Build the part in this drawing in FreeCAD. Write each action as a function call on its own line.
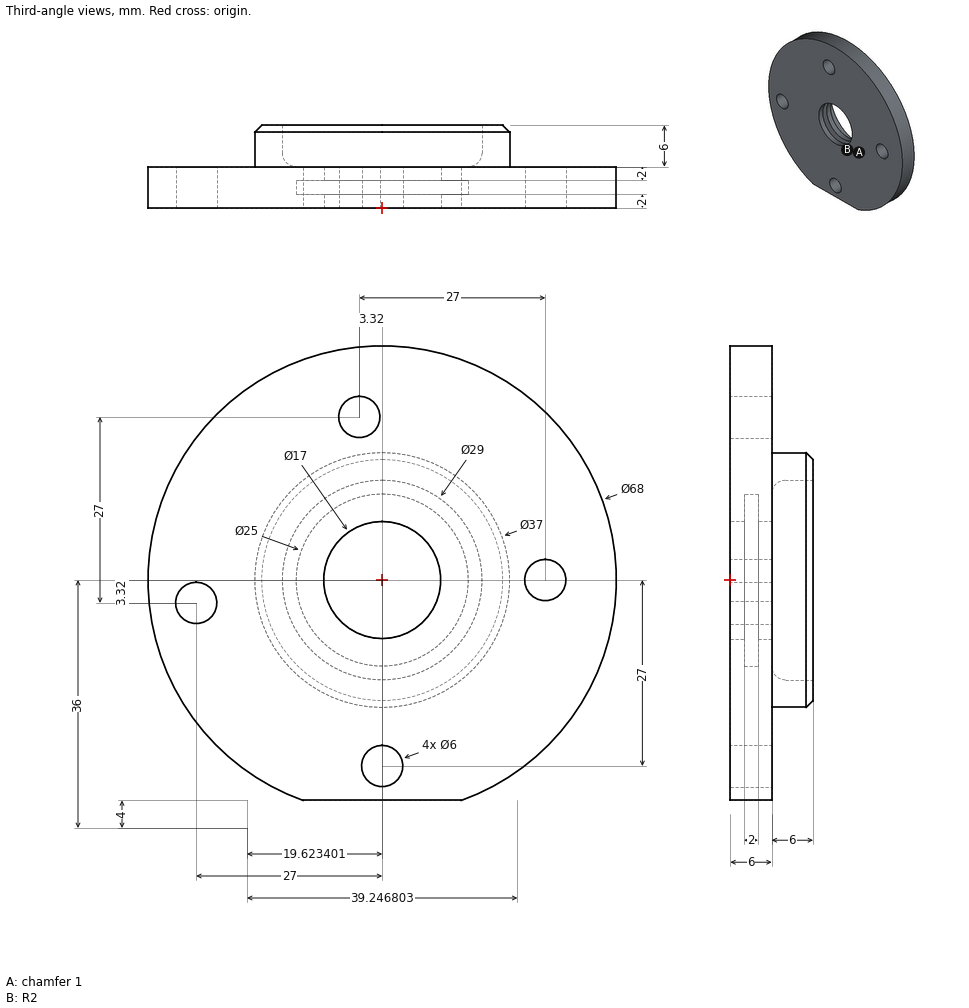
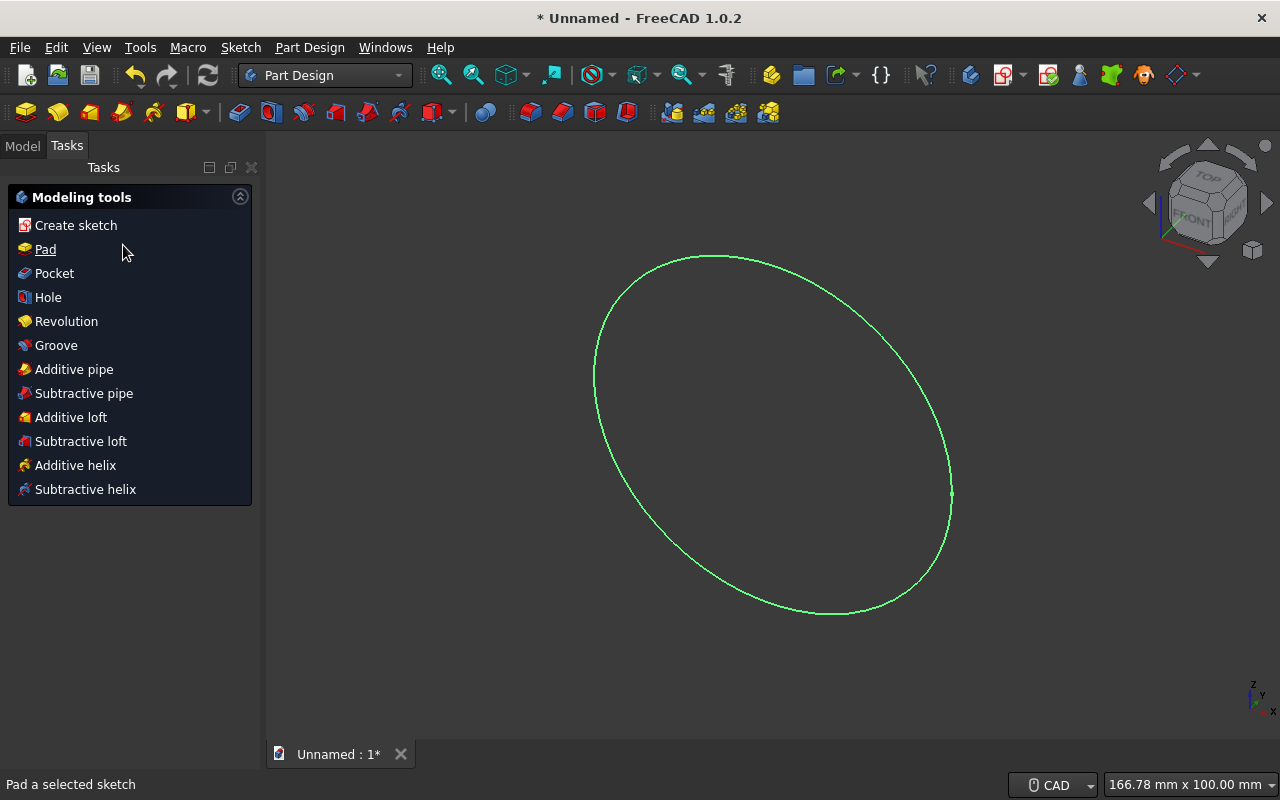
click(26, 112)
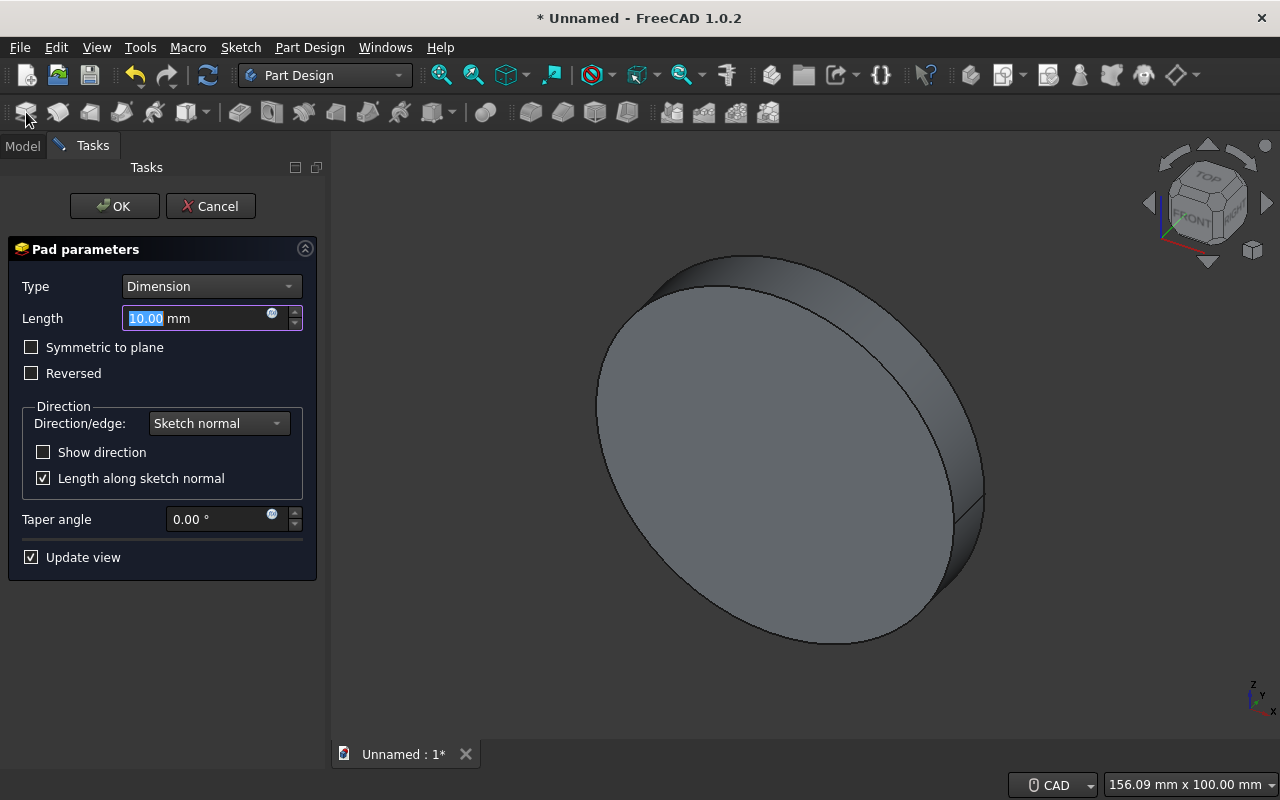
text(6)
key(Tab)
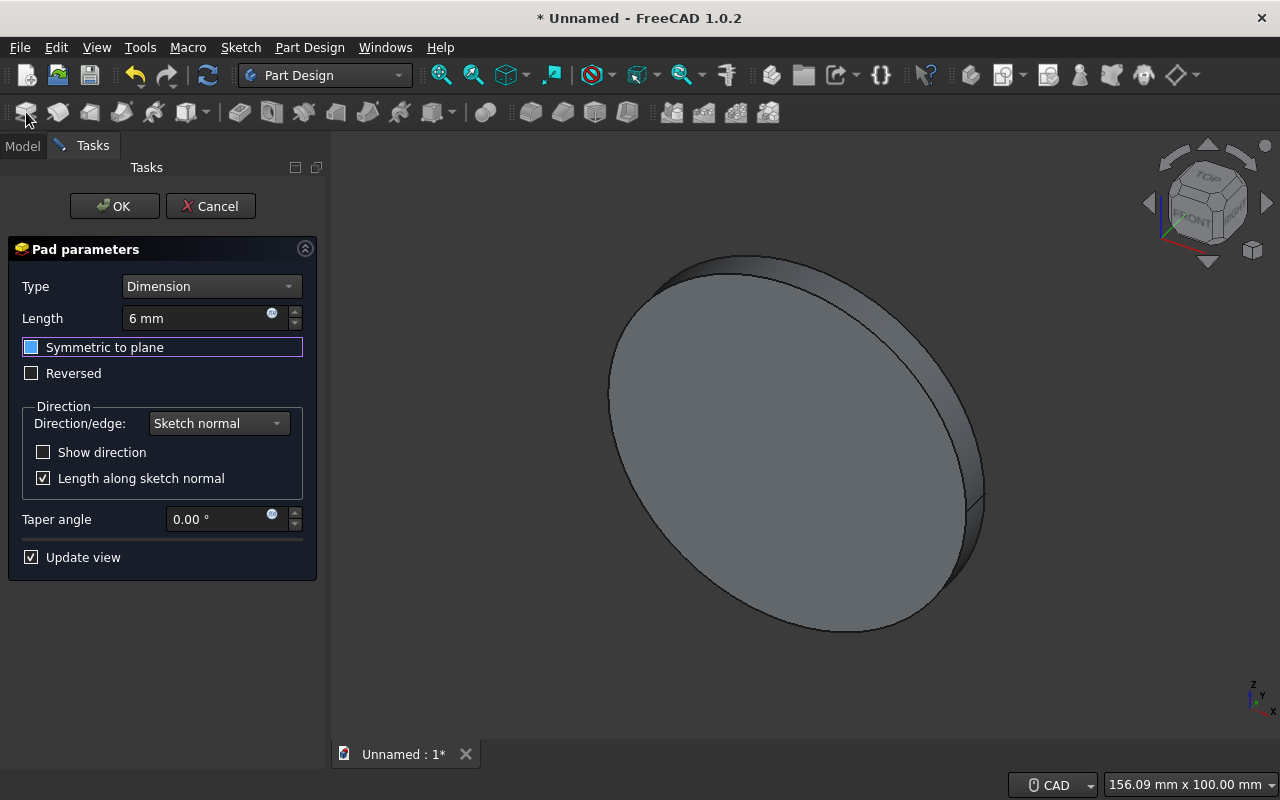
click(30, 373)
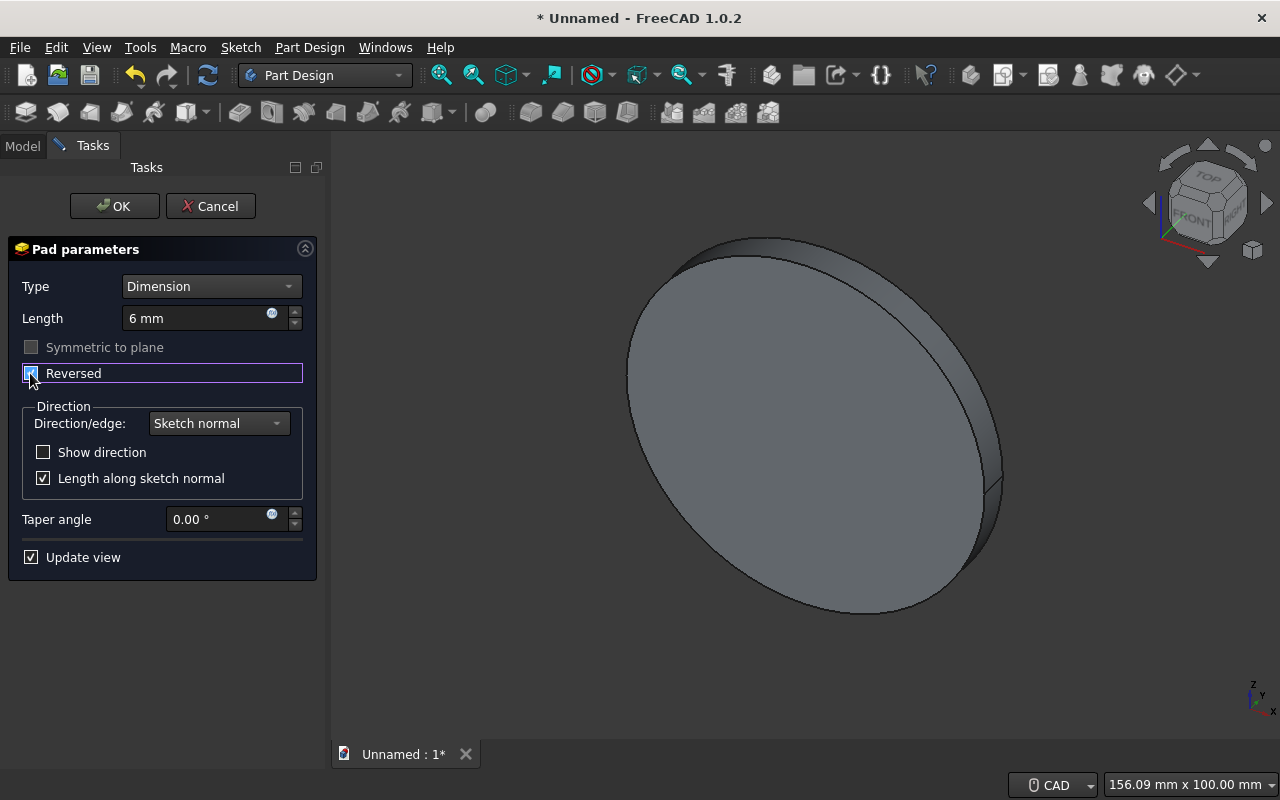
click(115, 206)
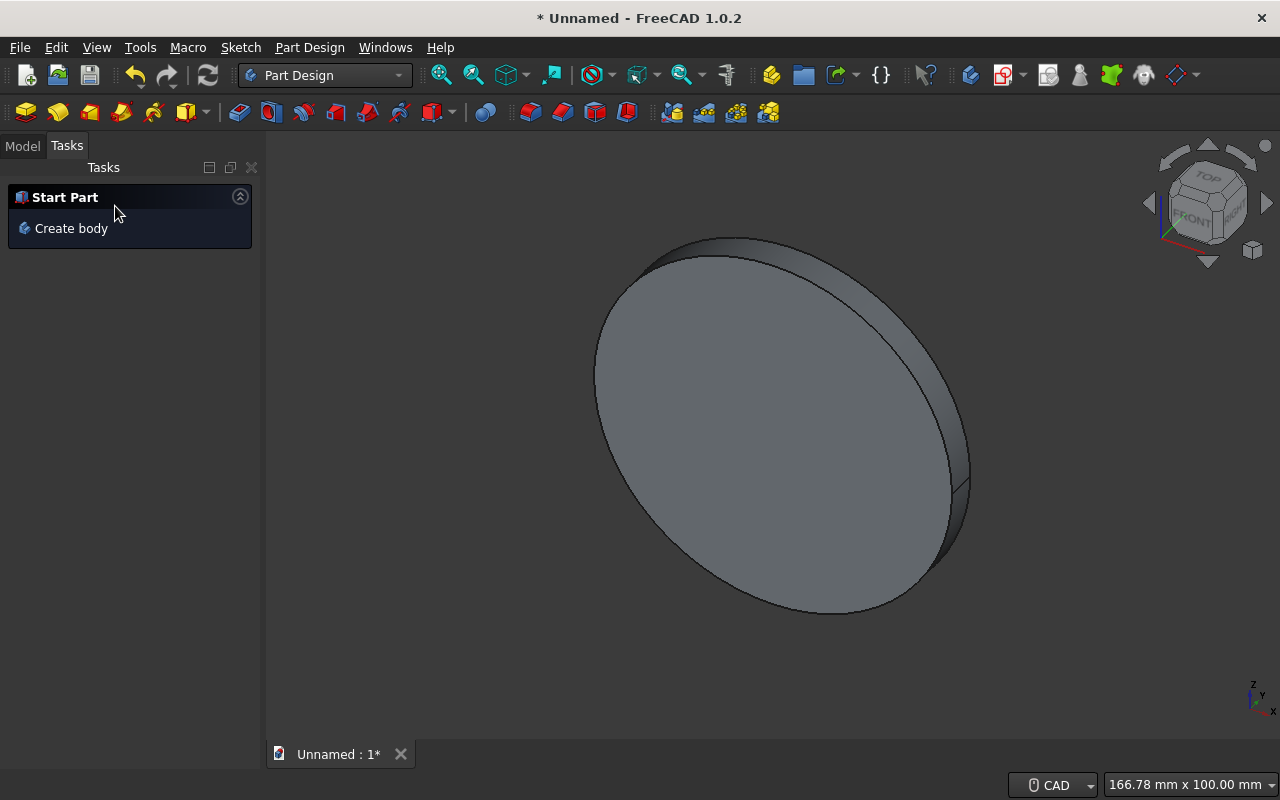
key(4)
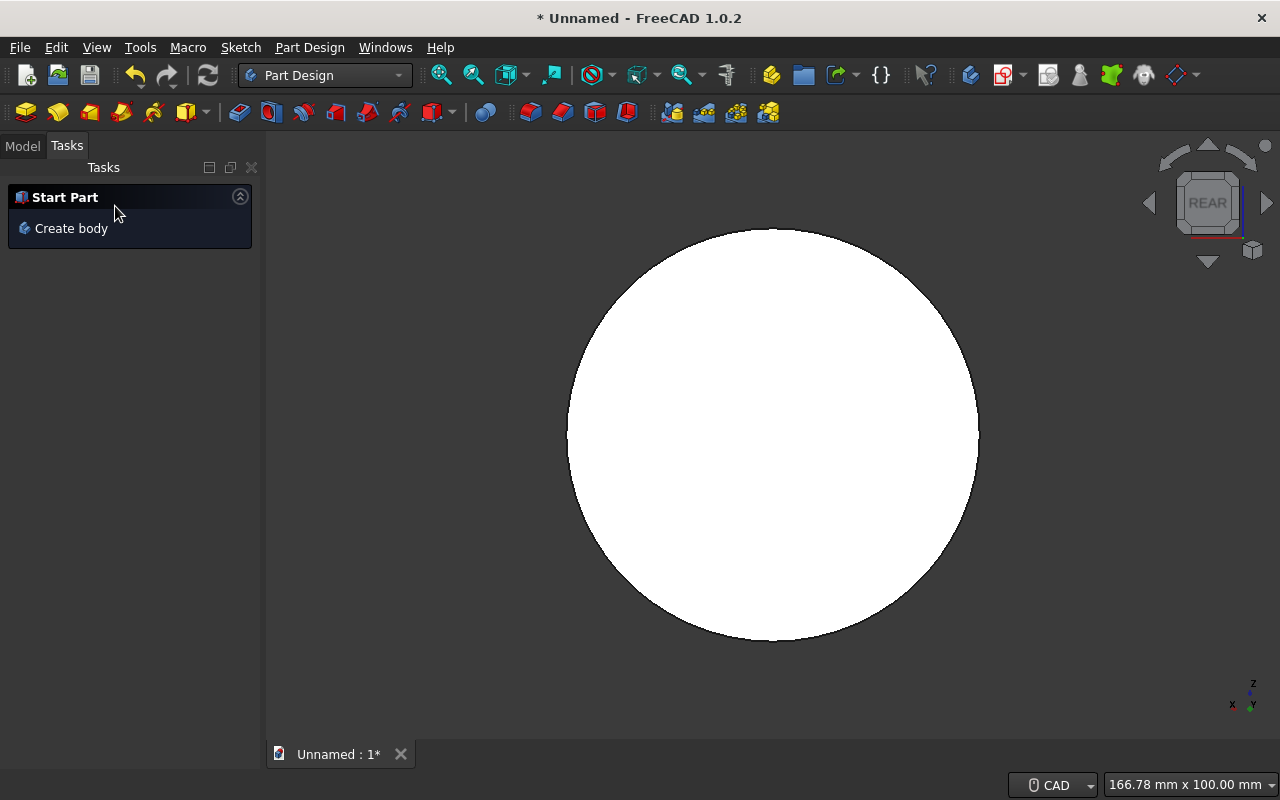
click(773, 434)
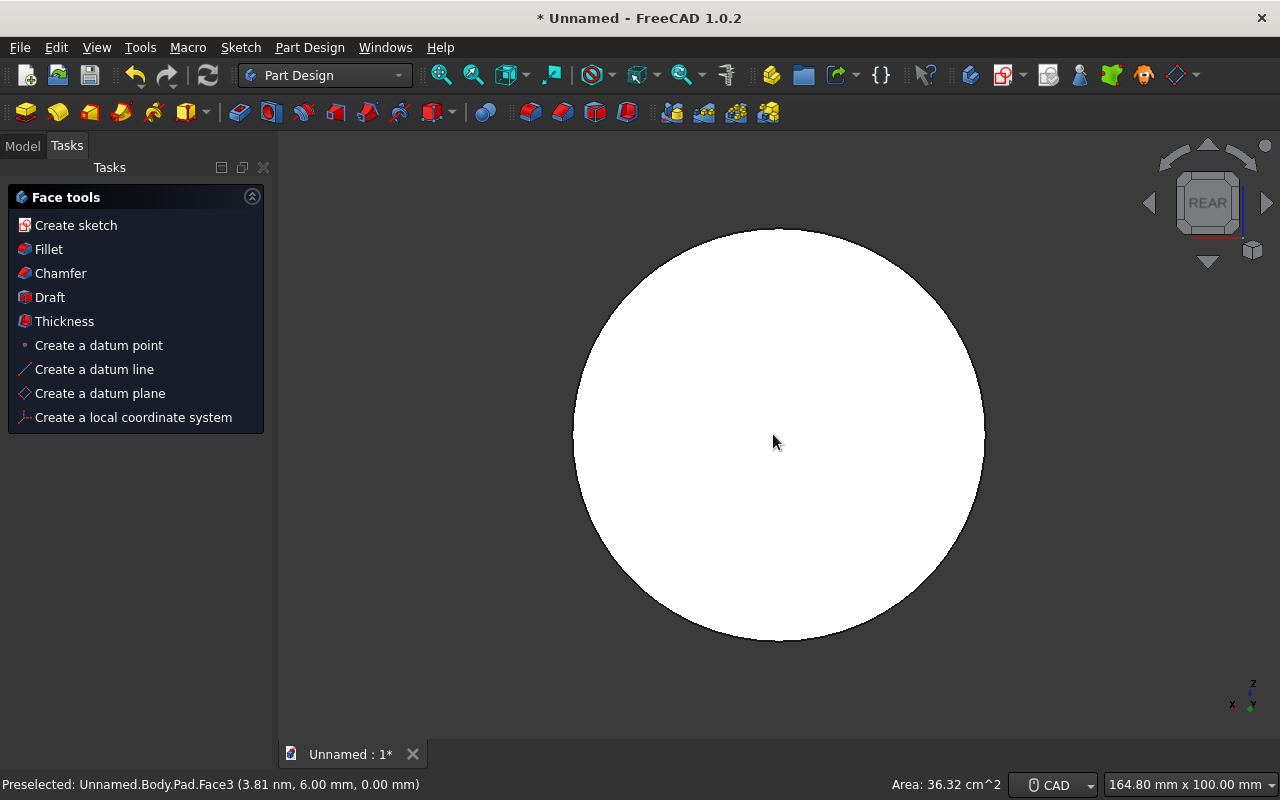
click(1004, 76)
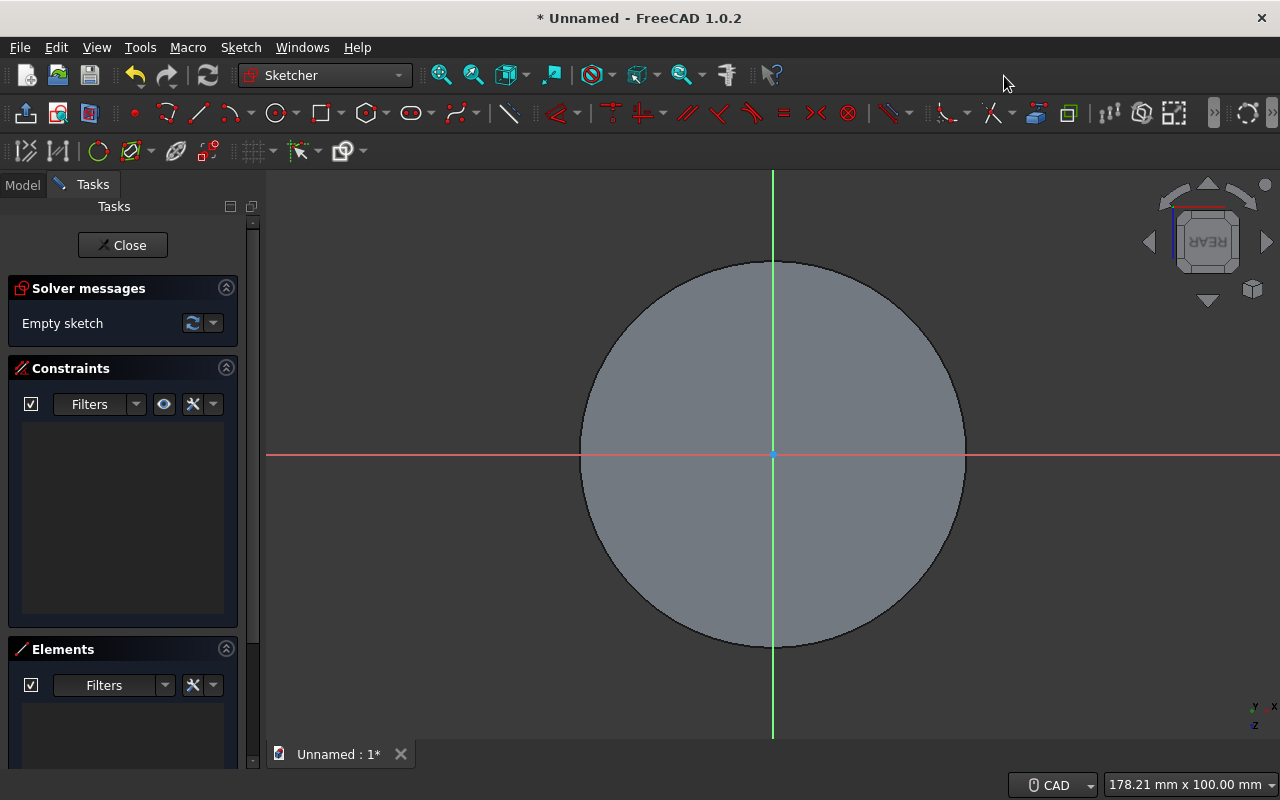
scroll(856, 455, up, 3)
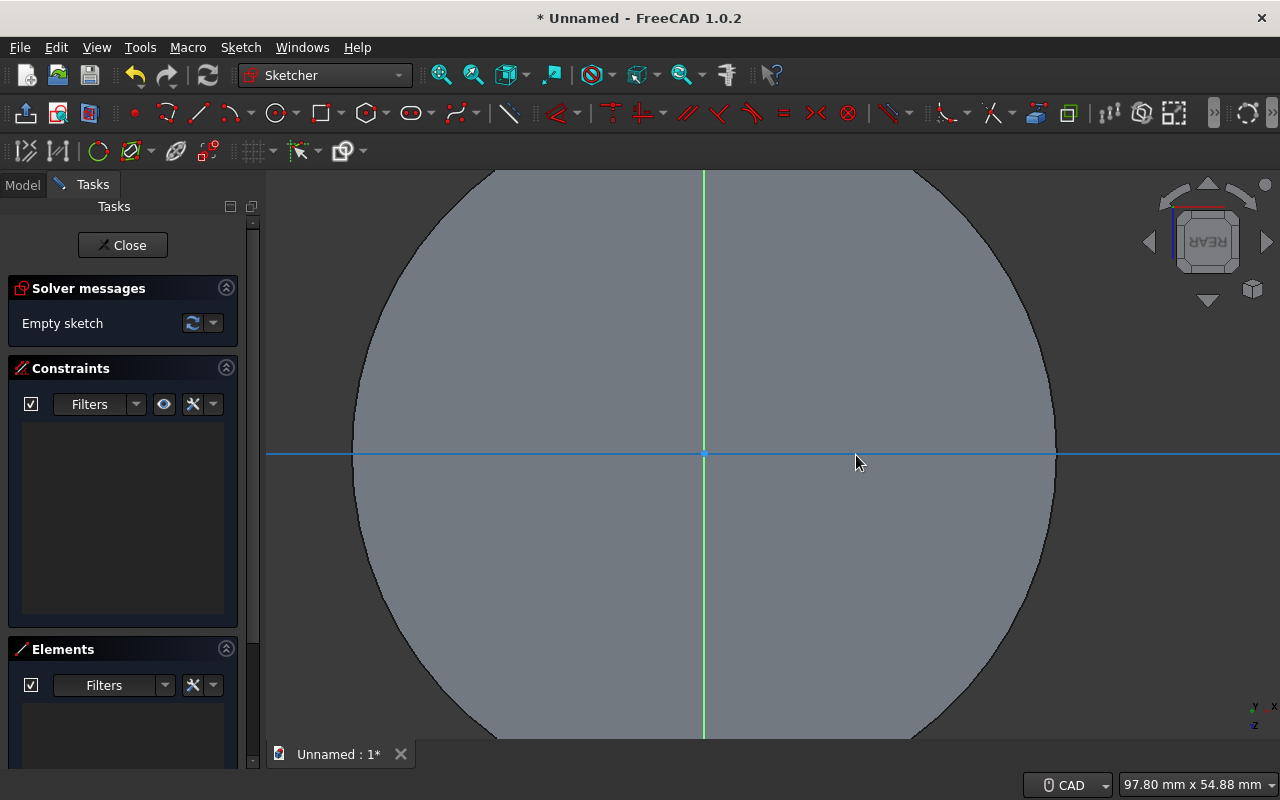
click(276, 114)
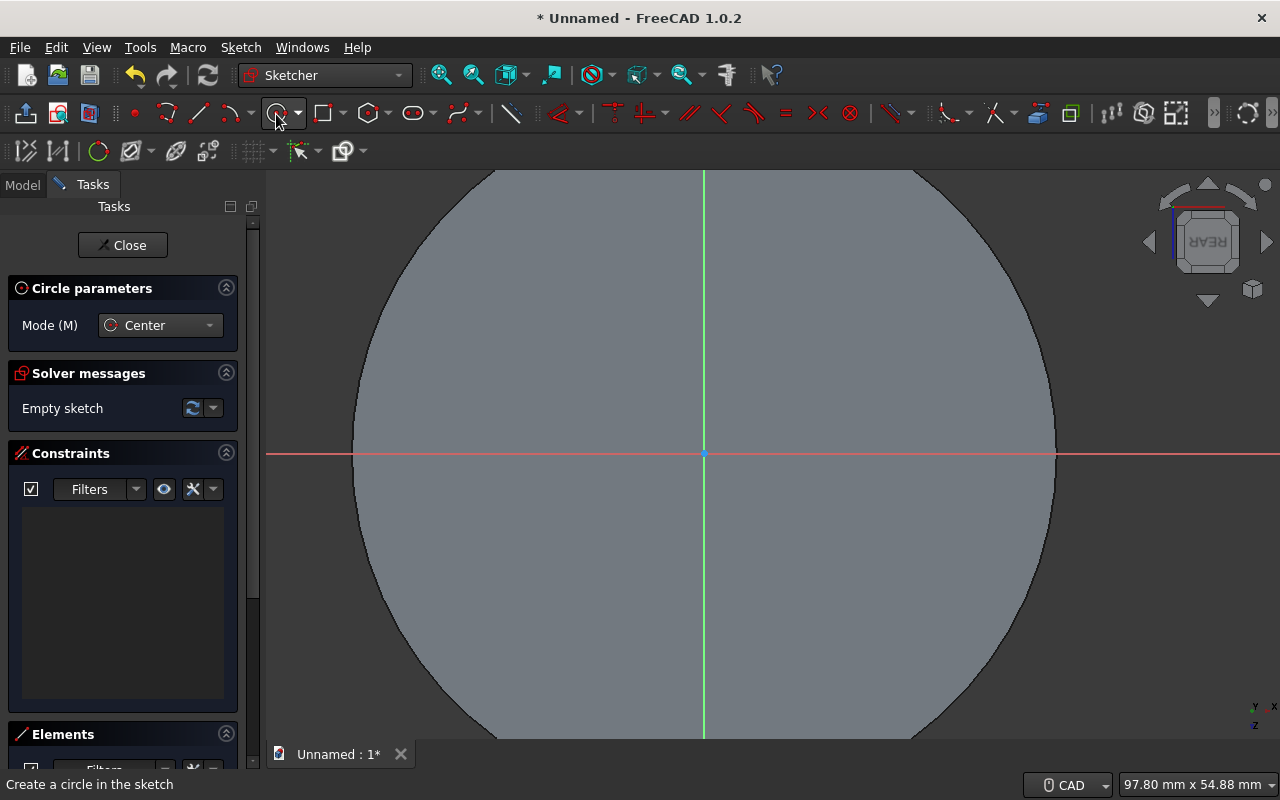
click(704, 454)
click(840, 318)
key(Escape)